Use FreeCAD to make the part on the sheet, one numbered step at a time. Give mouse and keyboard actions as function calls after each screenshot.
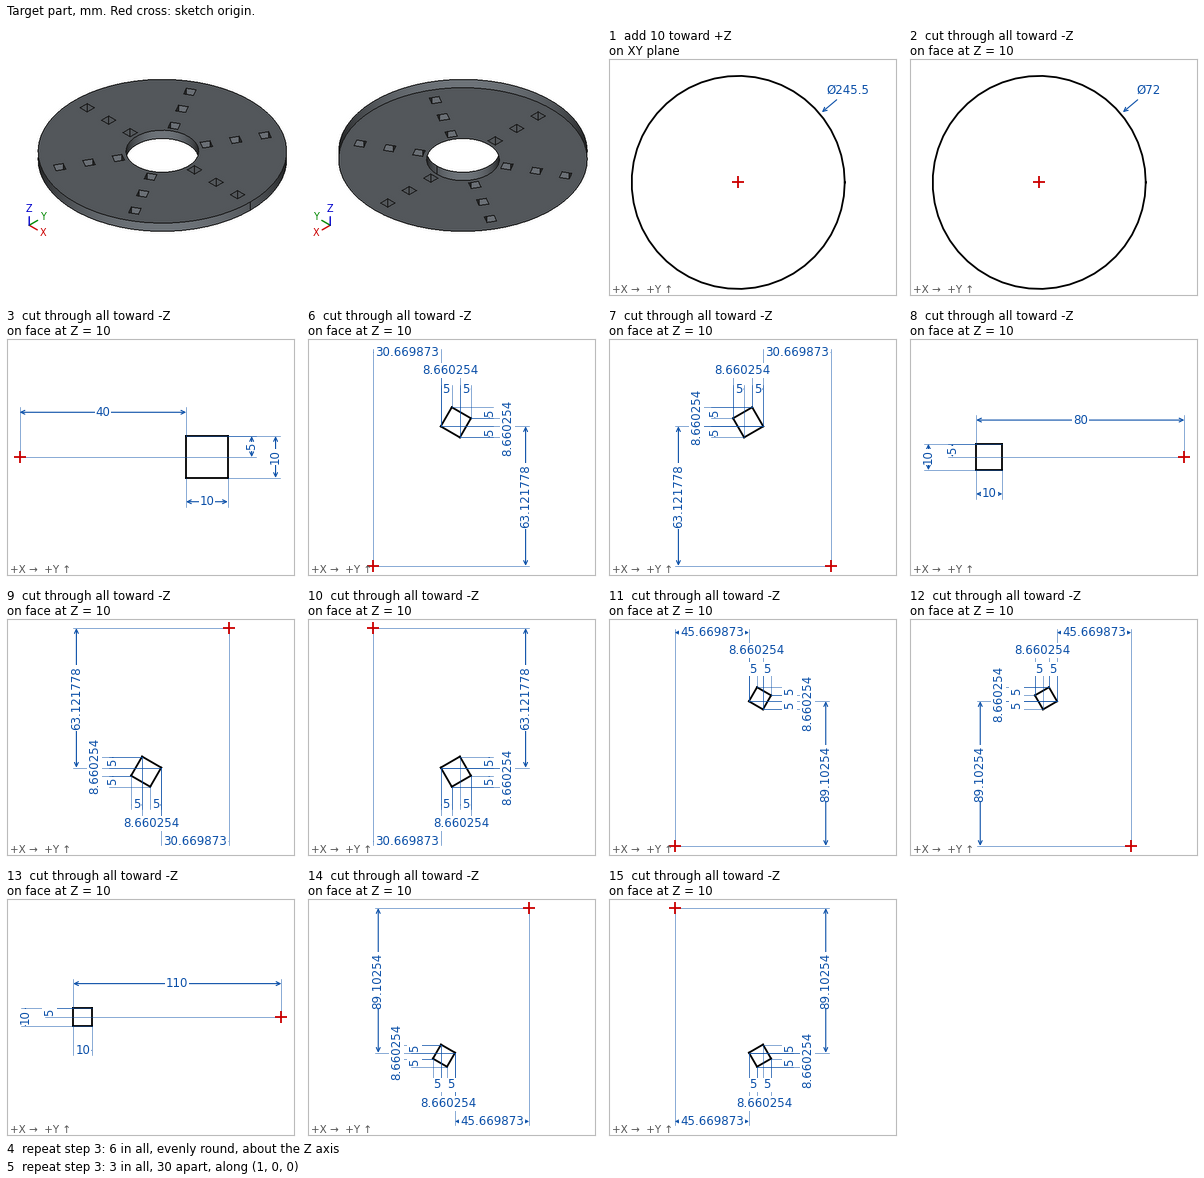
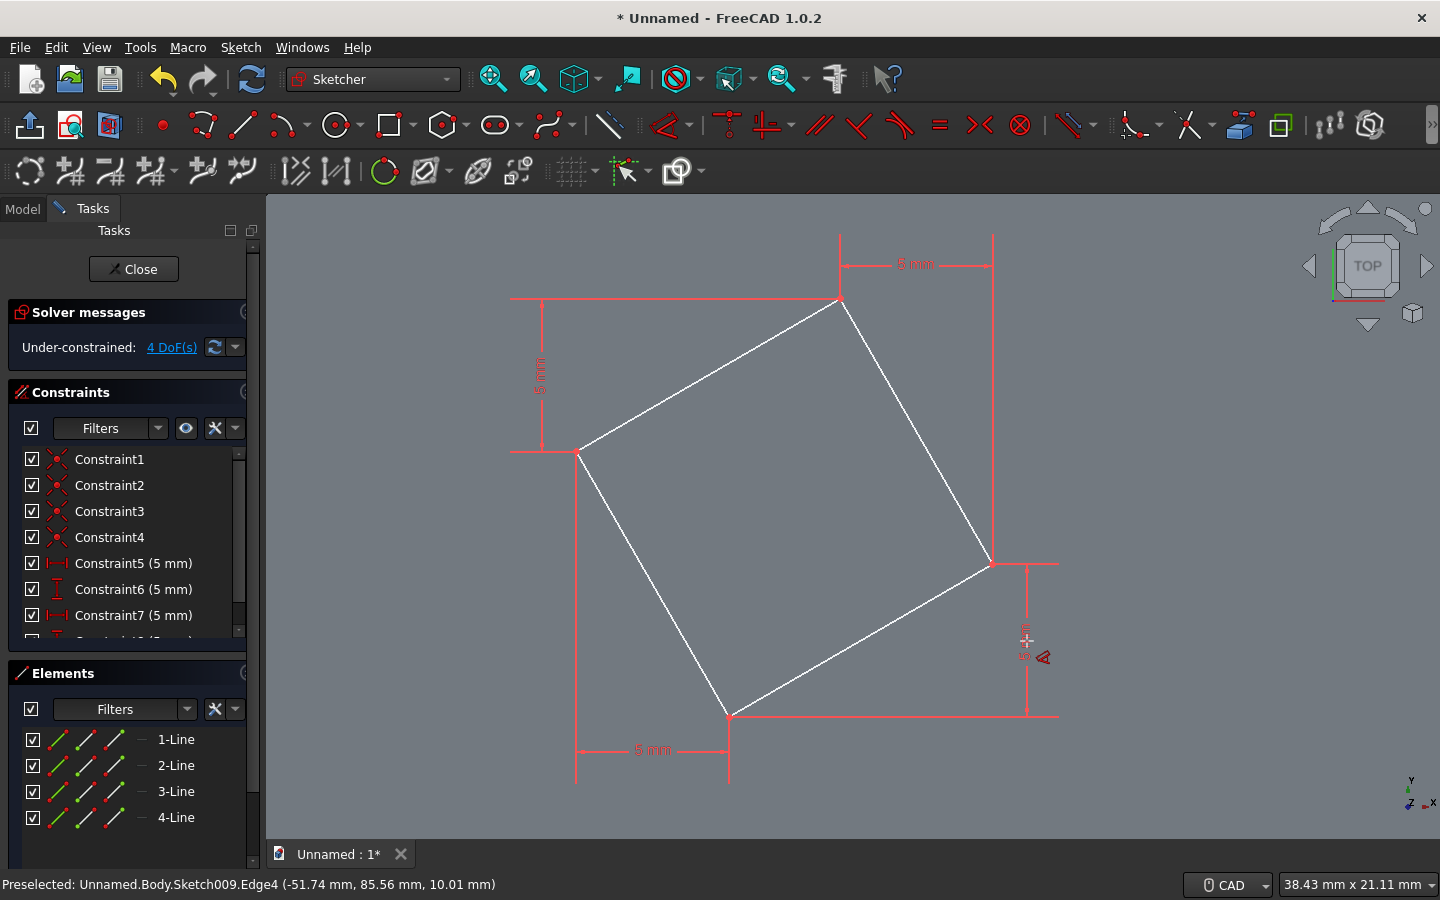
click(993, 564)
click(959, 688)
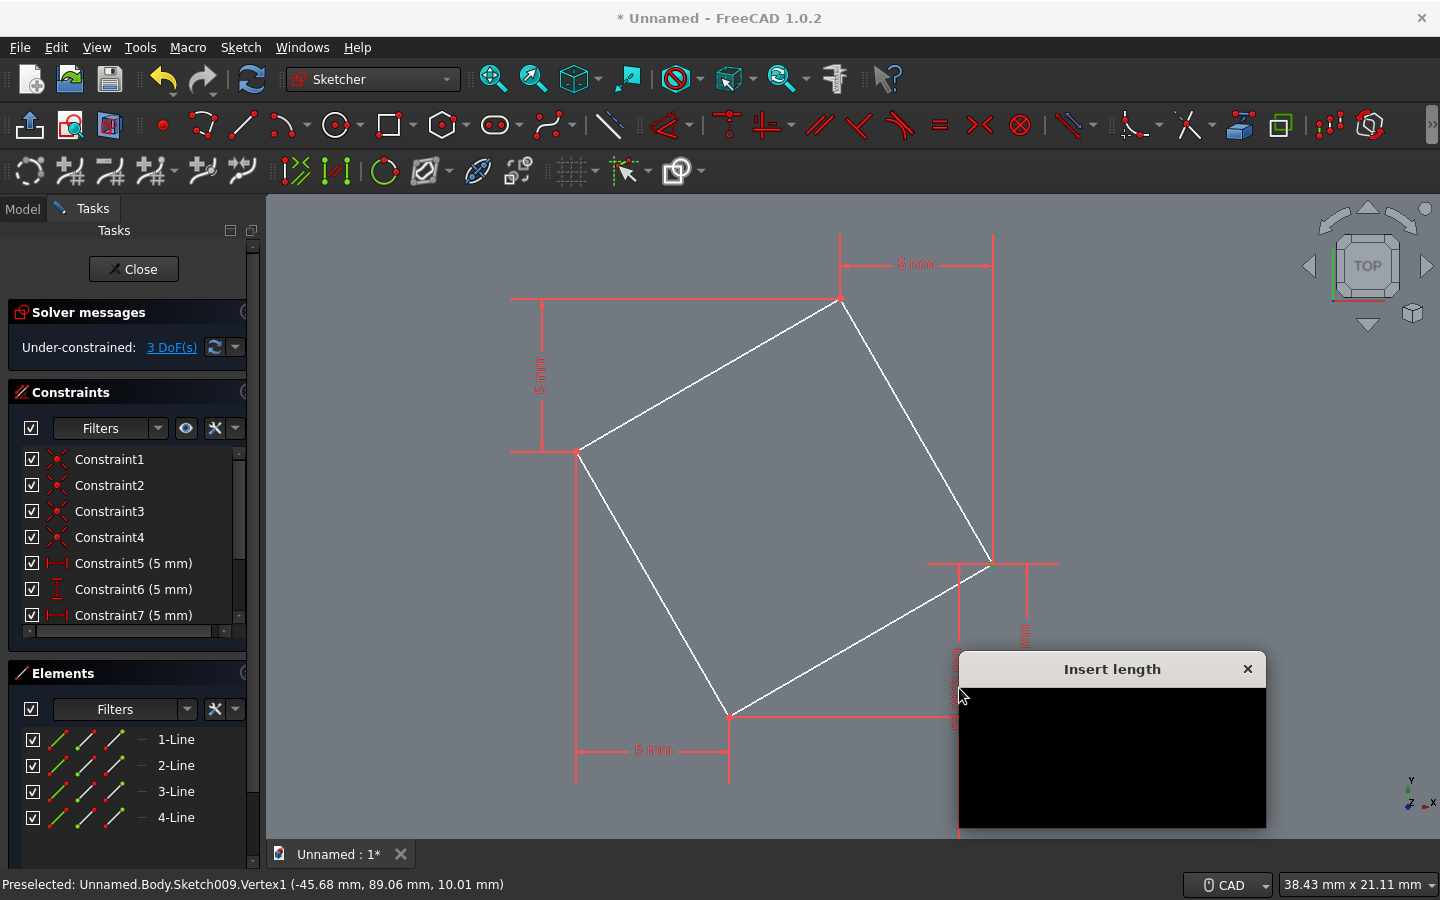
text(89.10254)
key(Return)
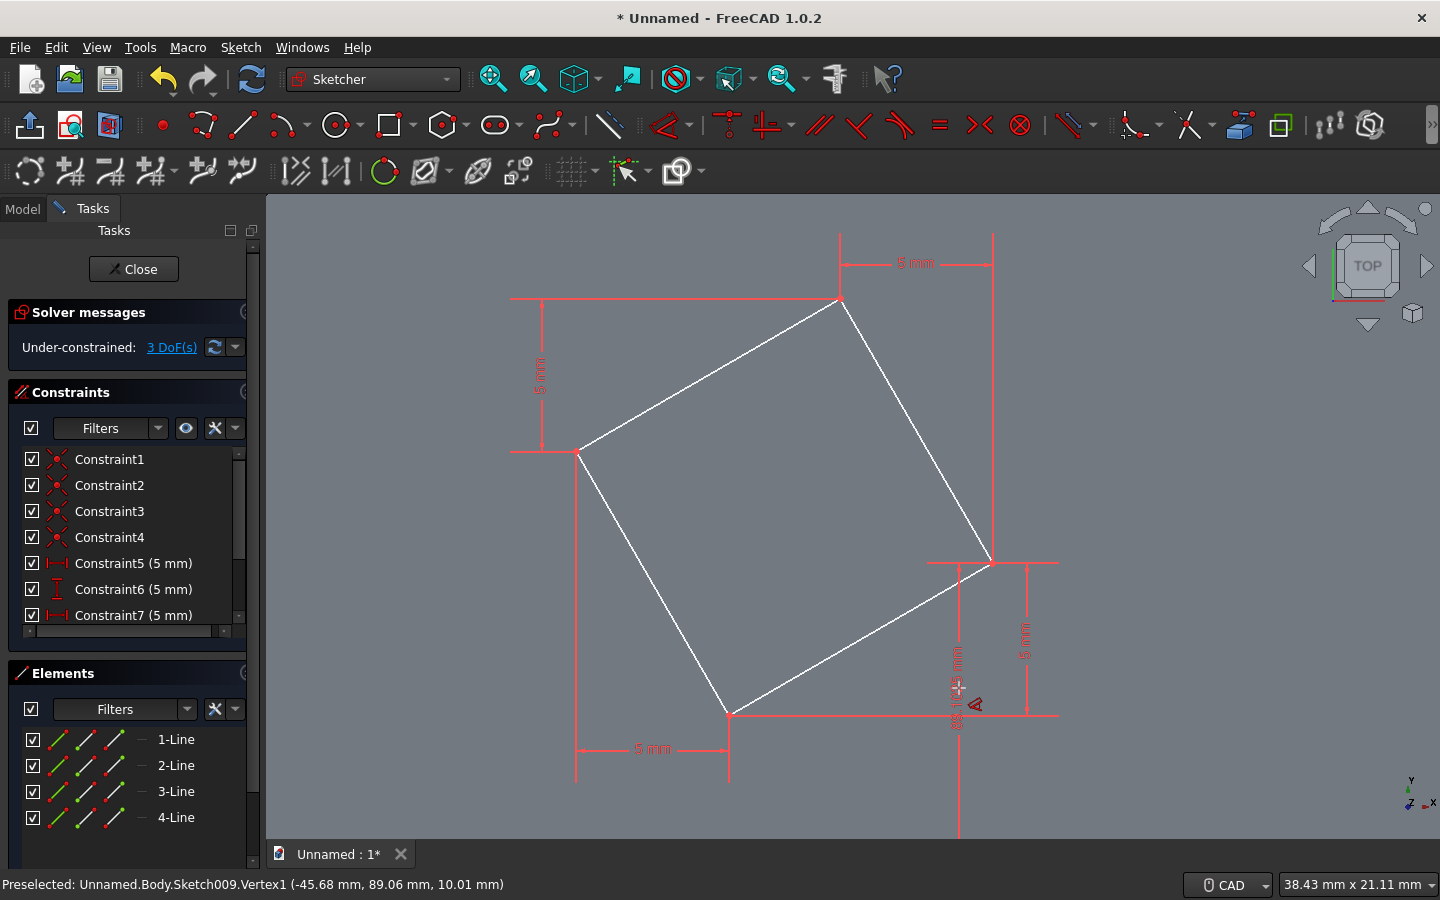
click(947, 484)
click(1027, 431)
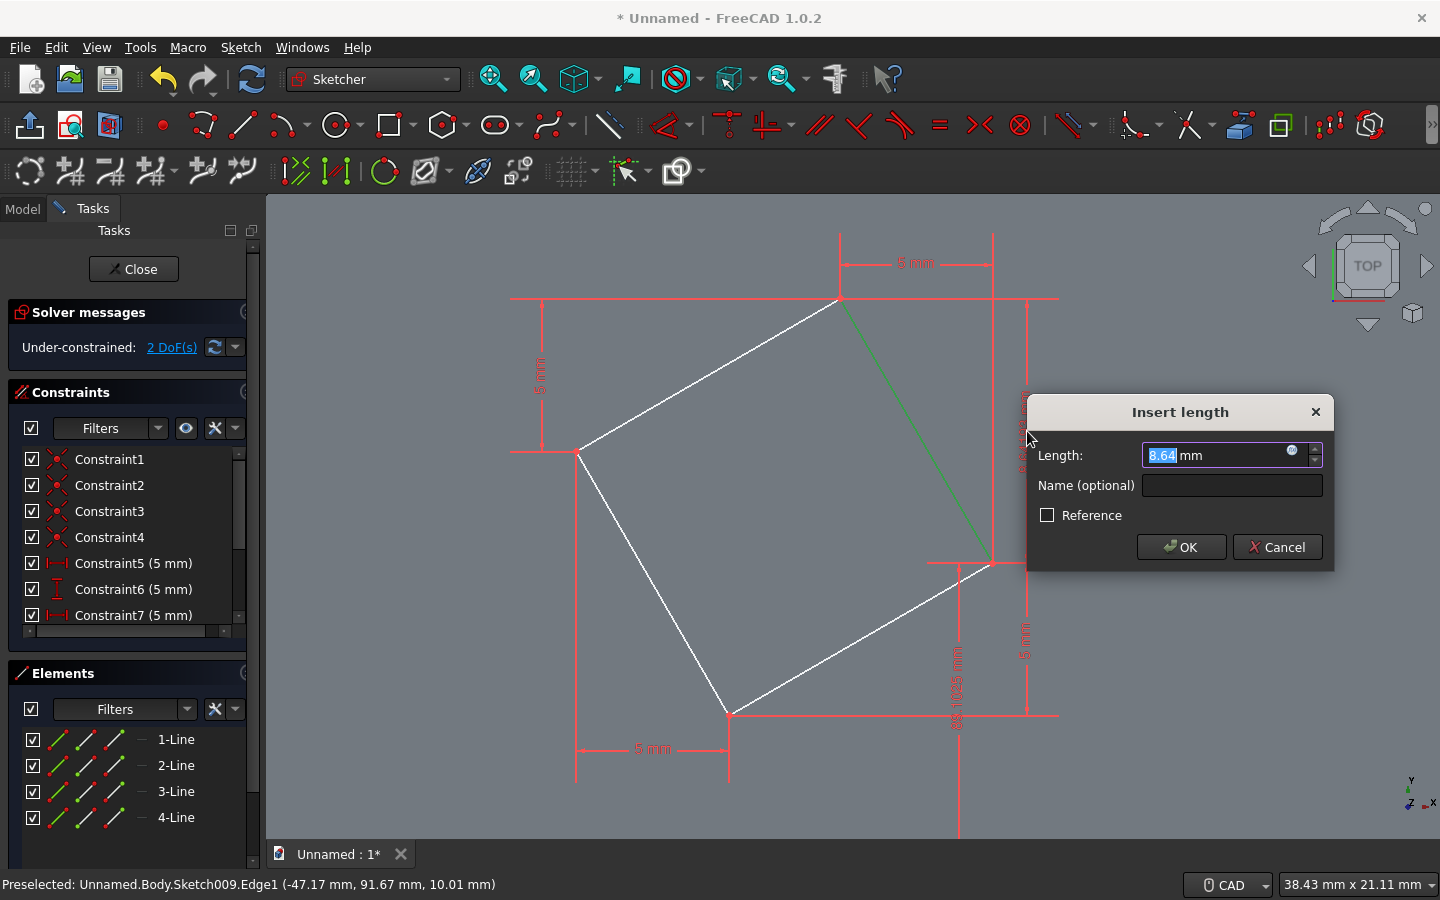
text(8.660254)
key(Return)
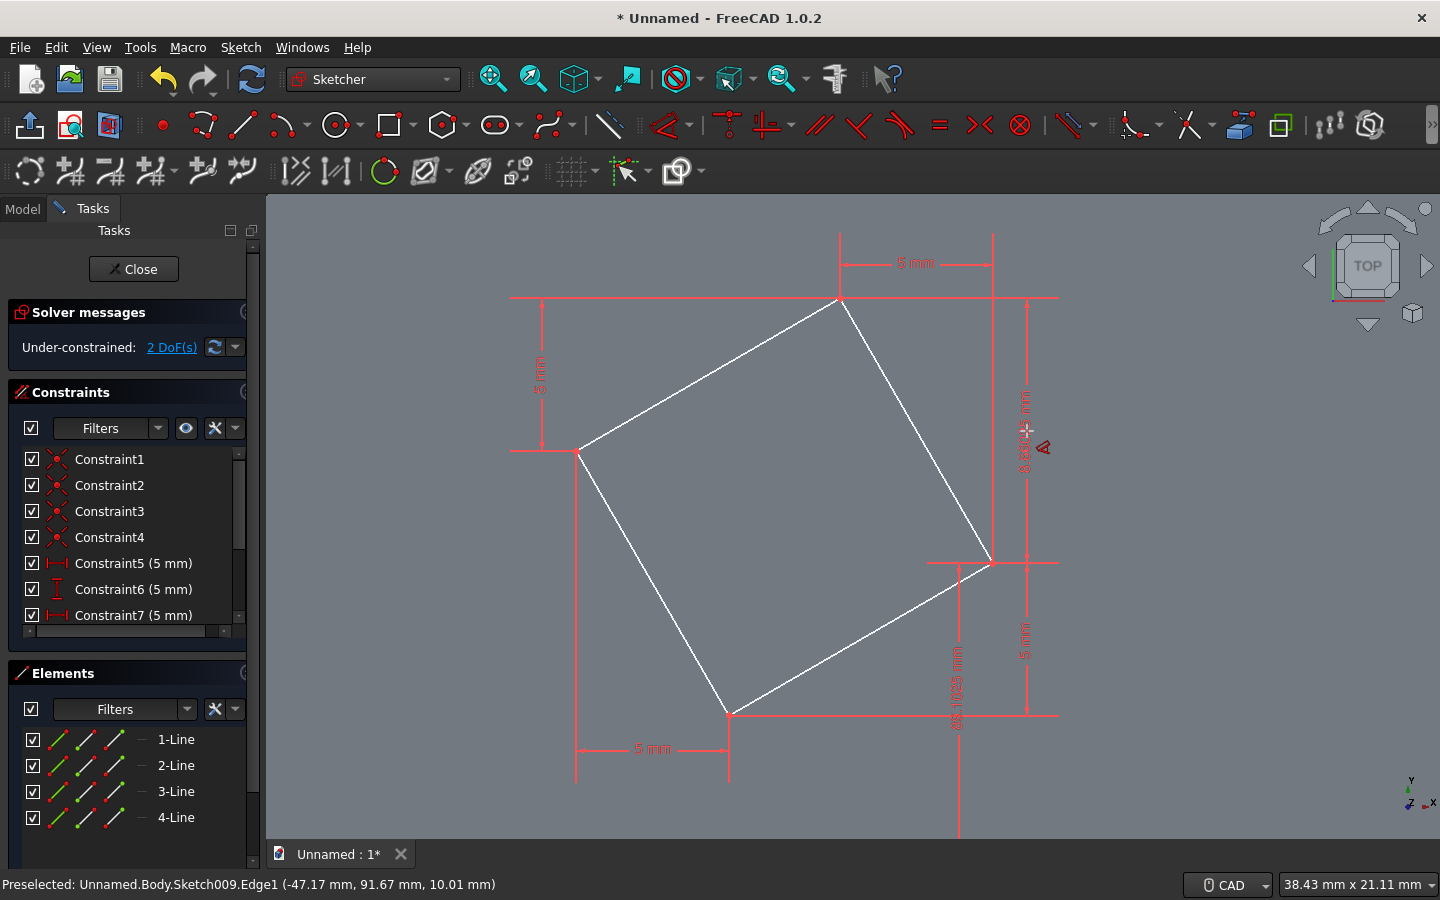
click(761, 344)
click(708, 264)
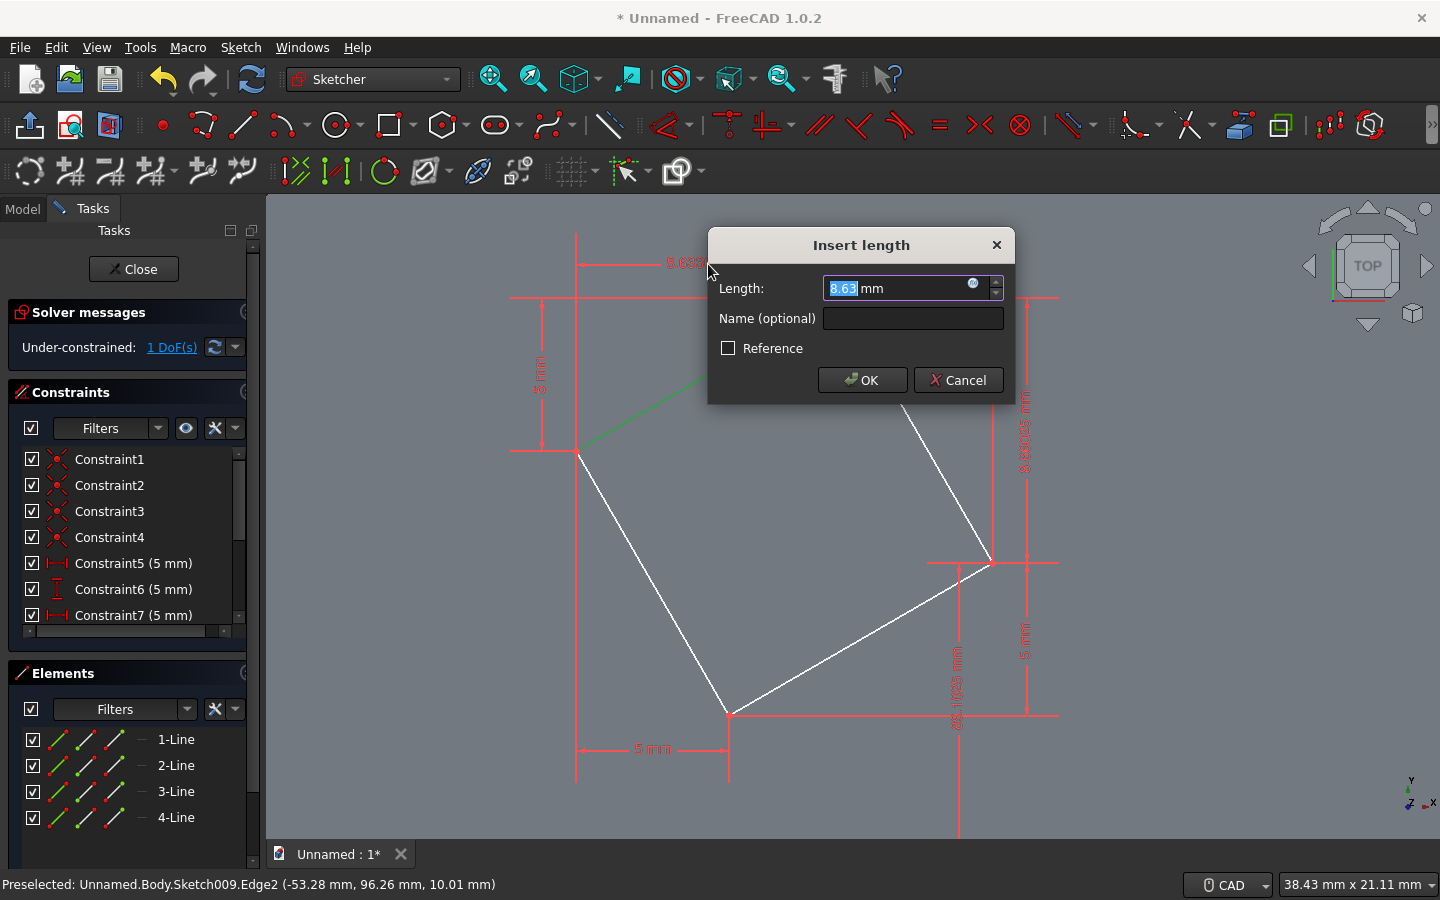
text(8.660254)
key(Return)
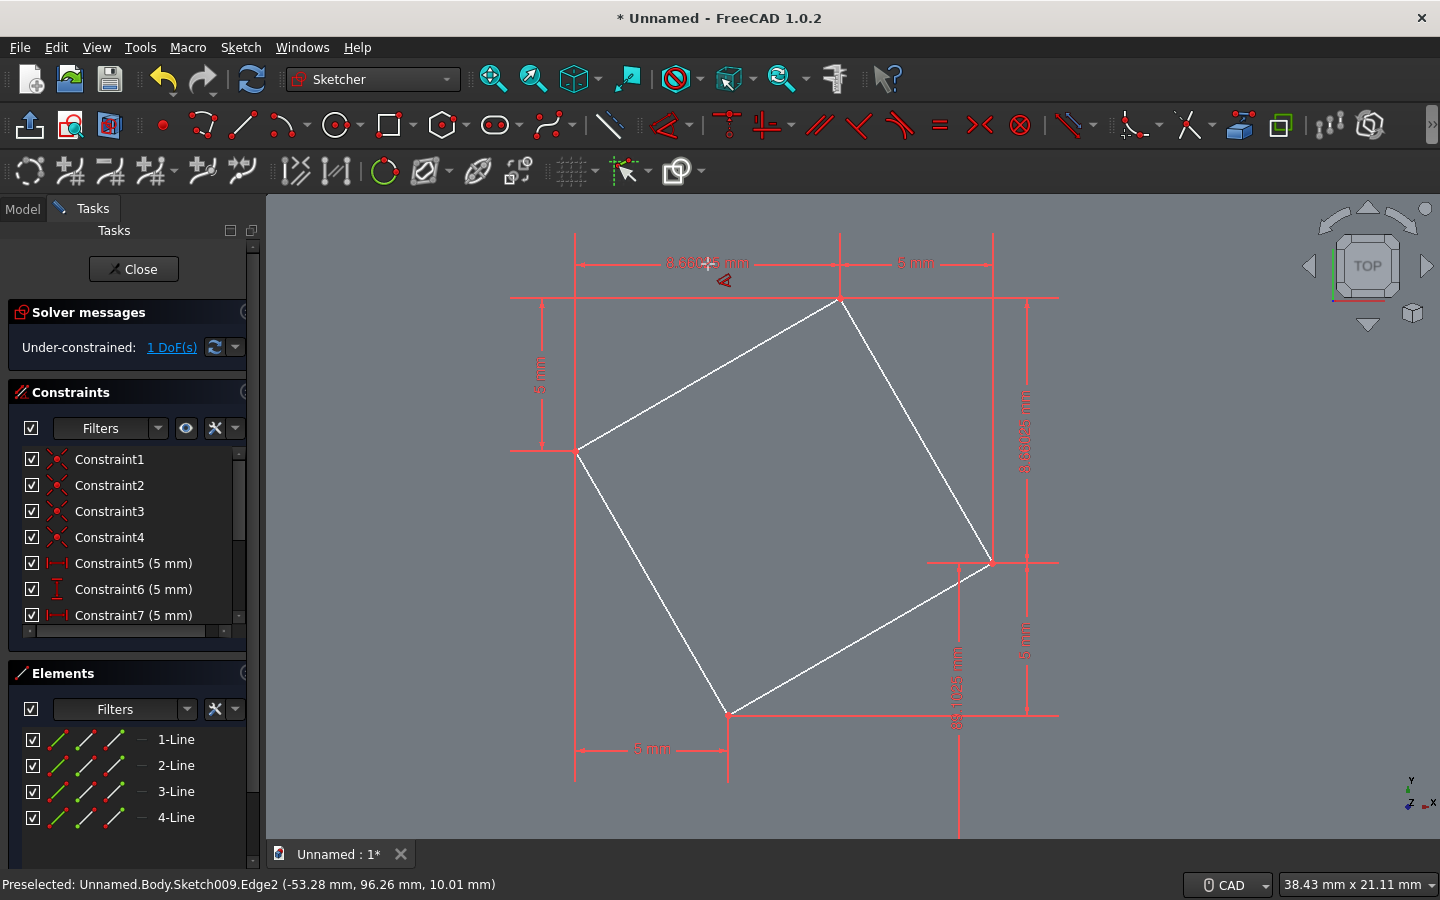
click(993, 563)
click(1134, 529)